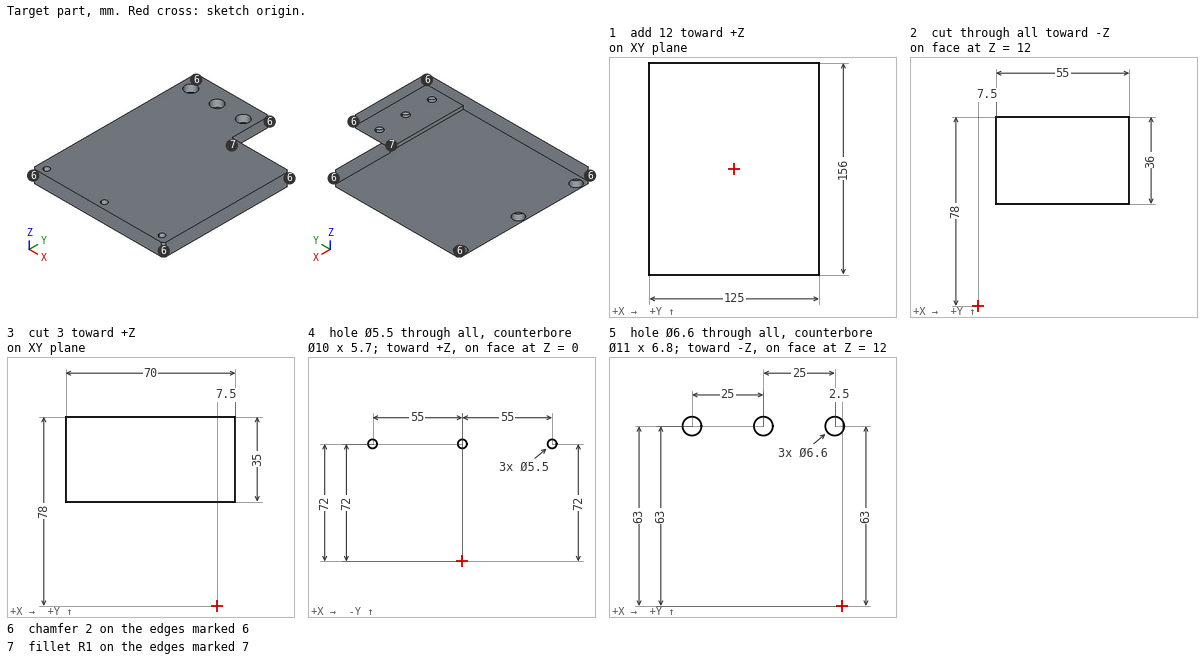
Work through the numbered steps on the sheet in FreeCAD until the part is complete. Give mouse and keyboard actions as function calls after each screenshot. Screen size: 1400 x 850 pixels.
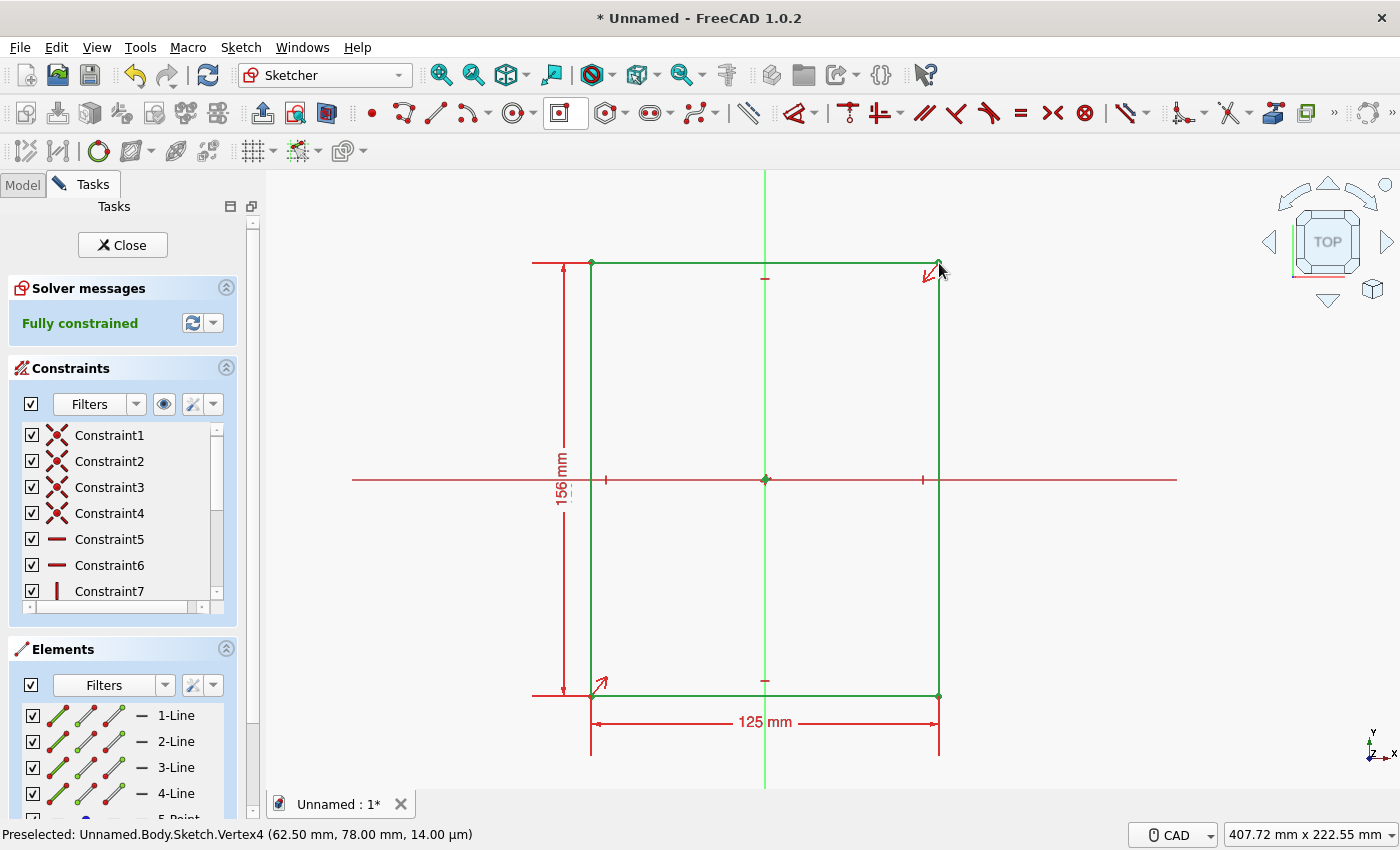
click(123, 245)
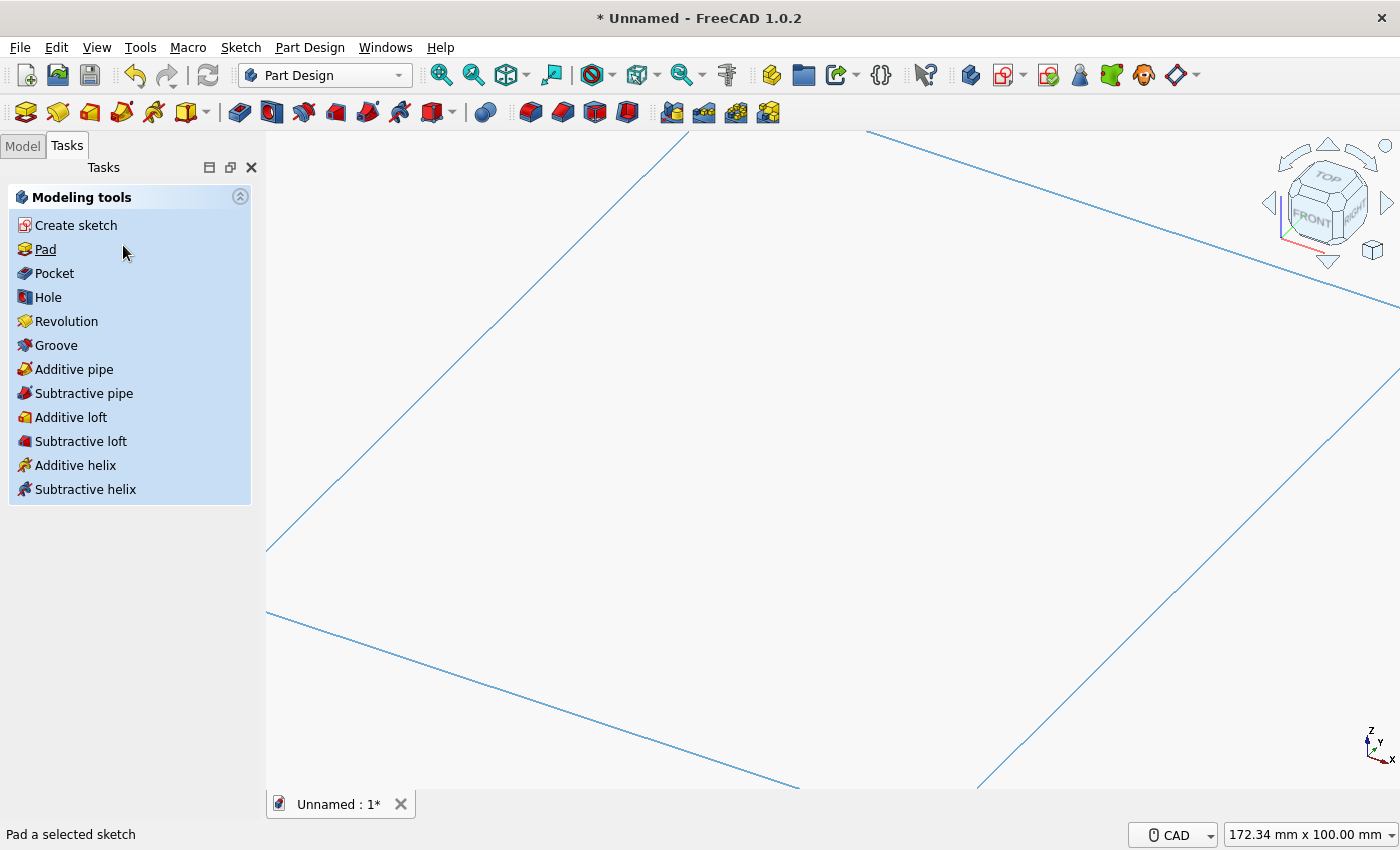
click(26, 112)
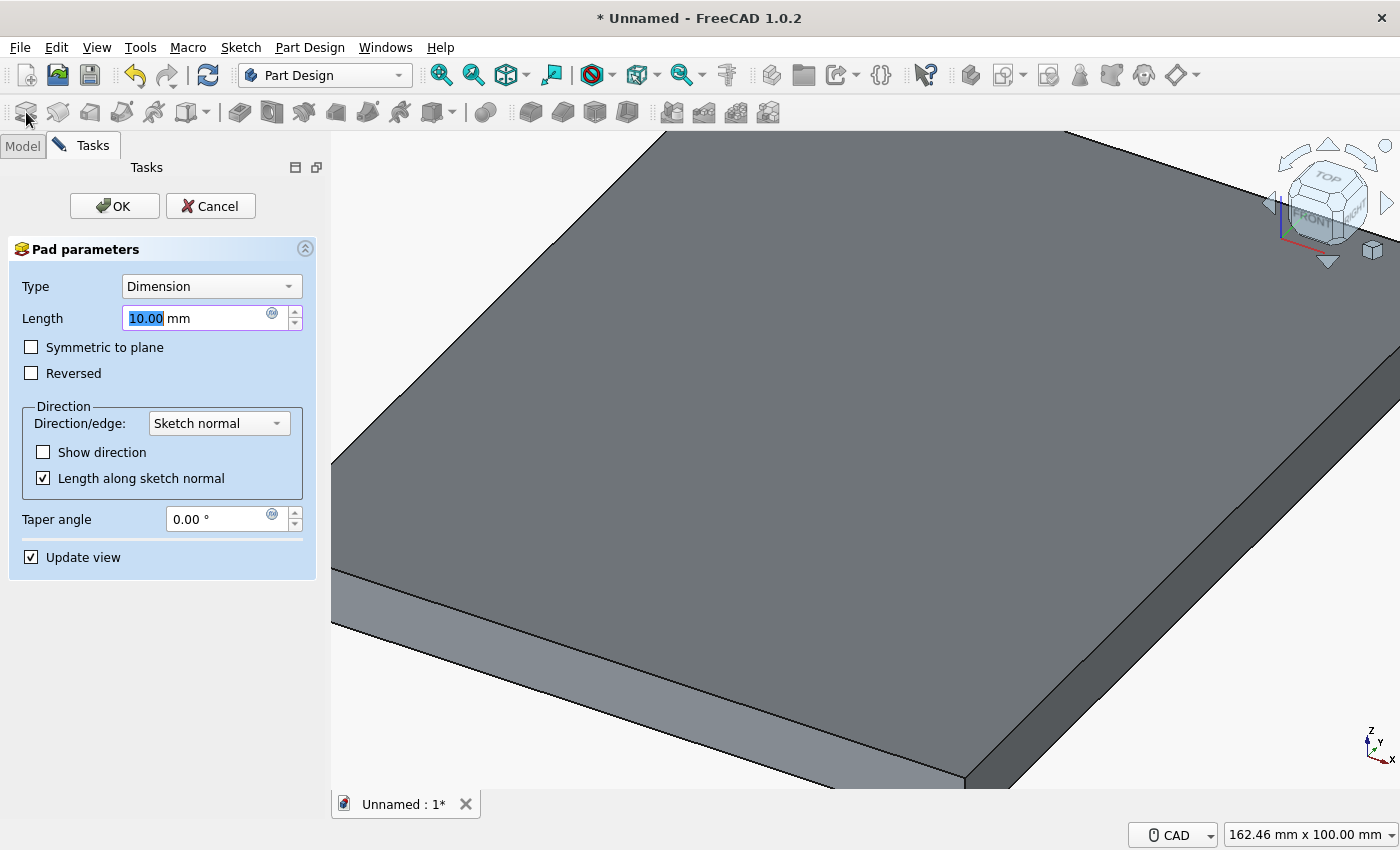
text(12)
key(Tab)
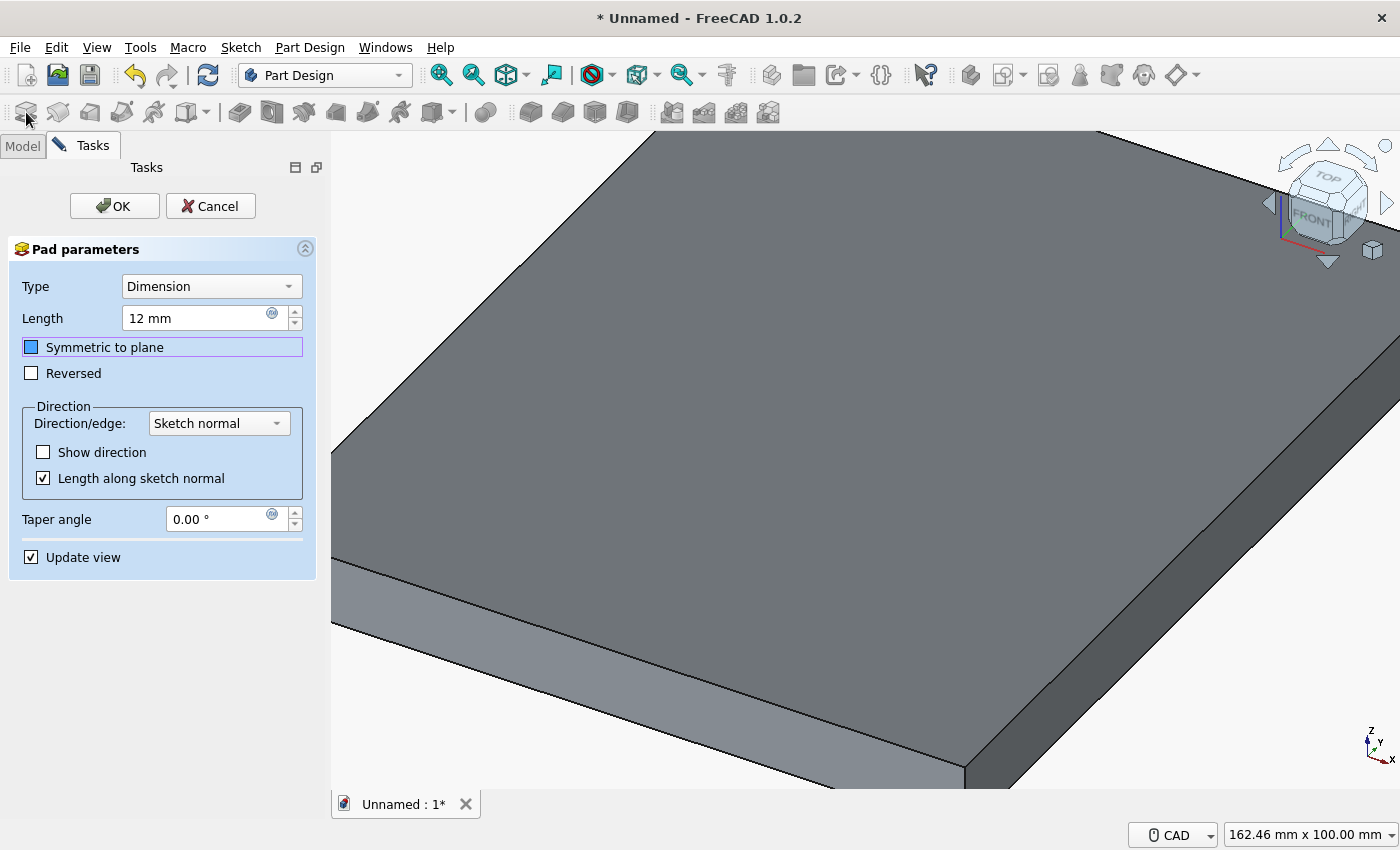
click(115, 206)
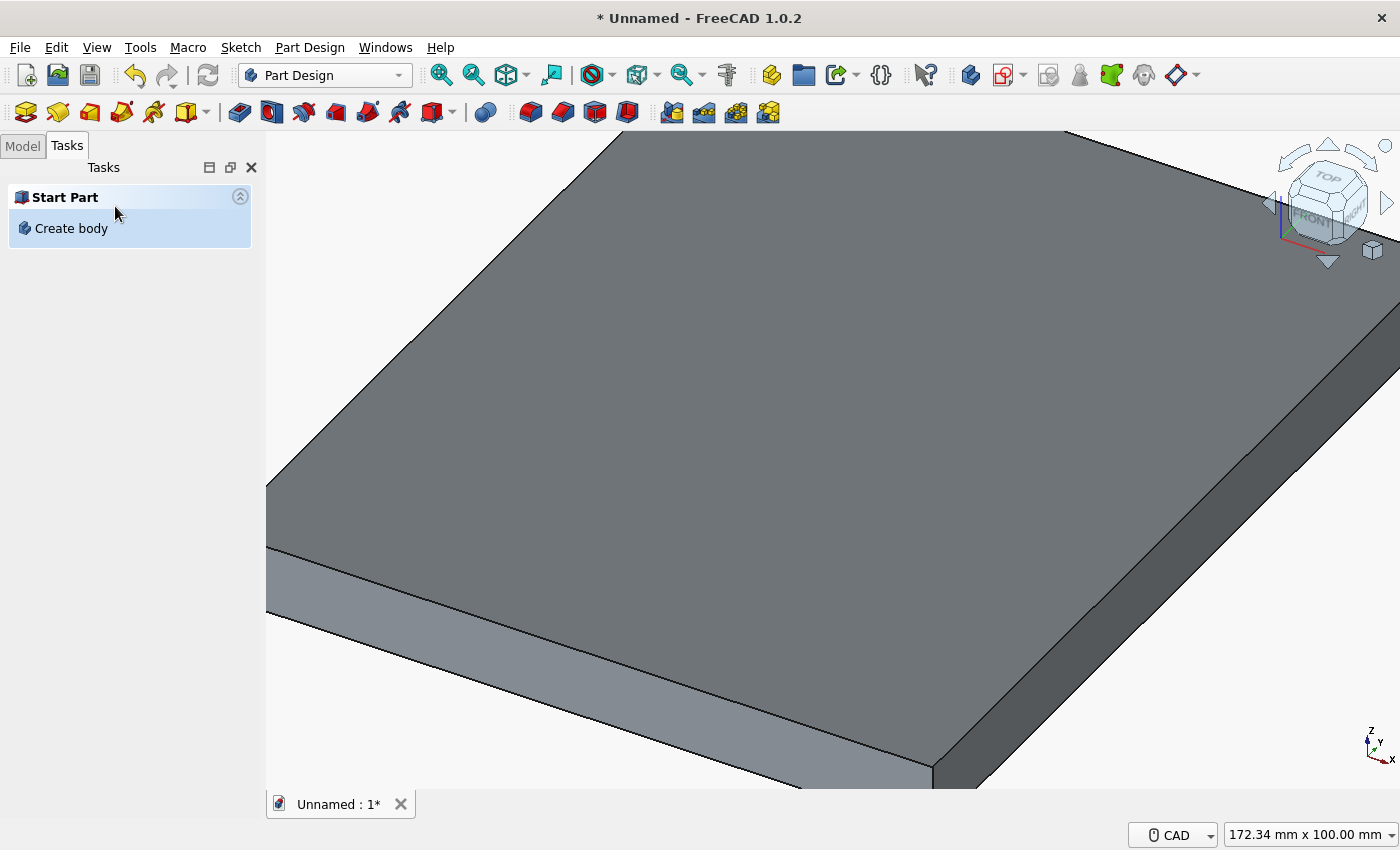
click(442, 76)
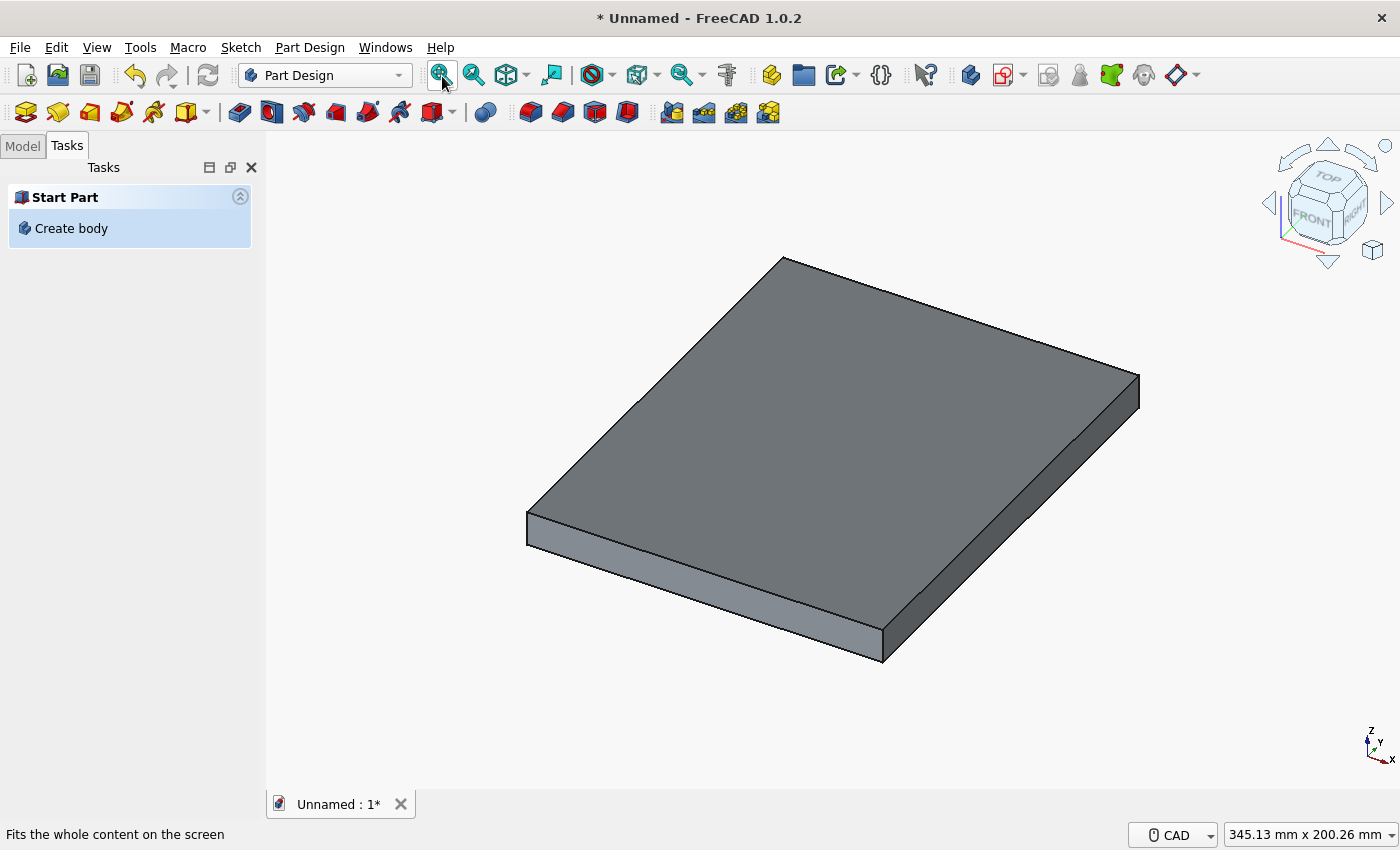
click(833, 443)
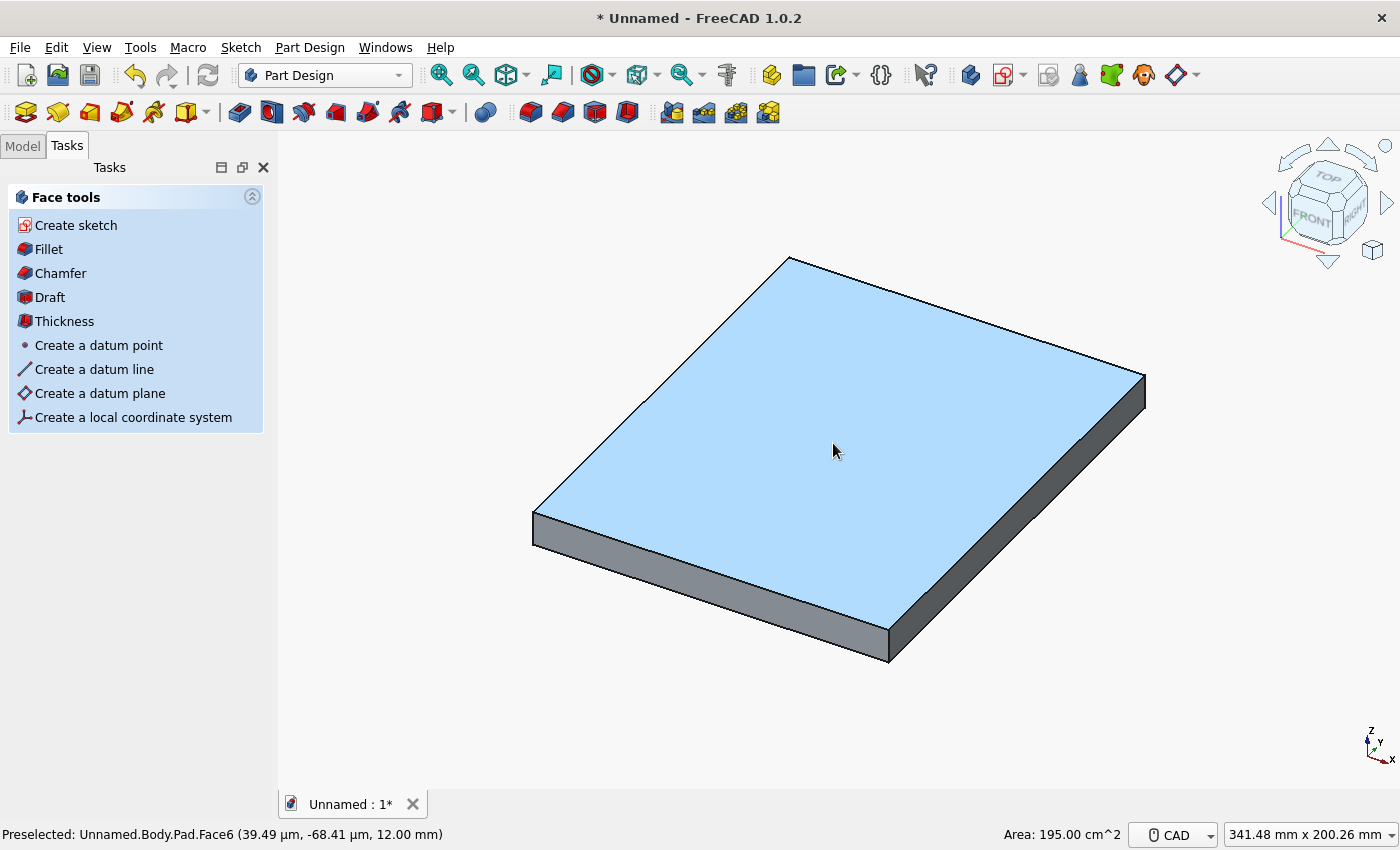
click(1004, 76)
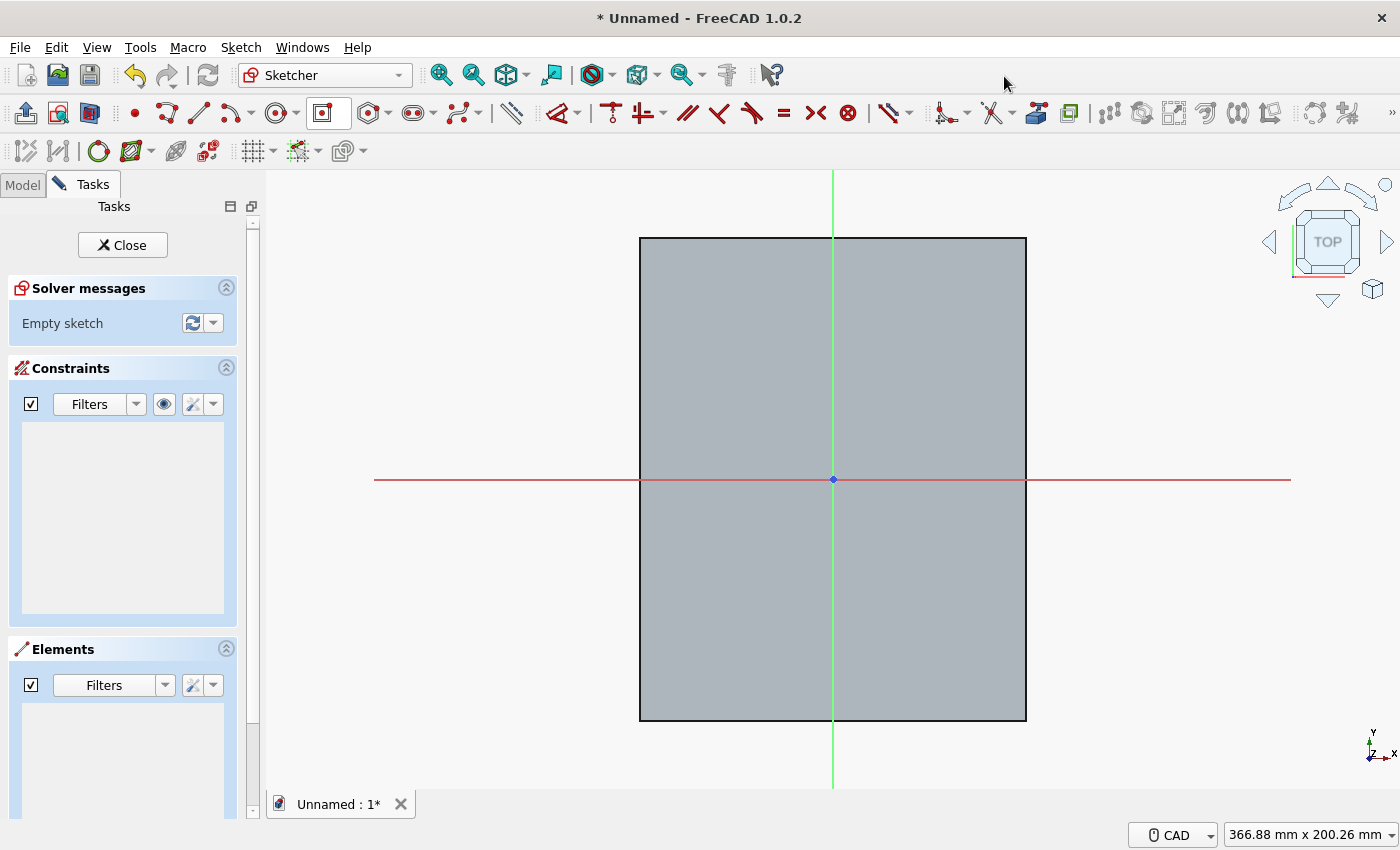
scroll(1235, 198, up, 2)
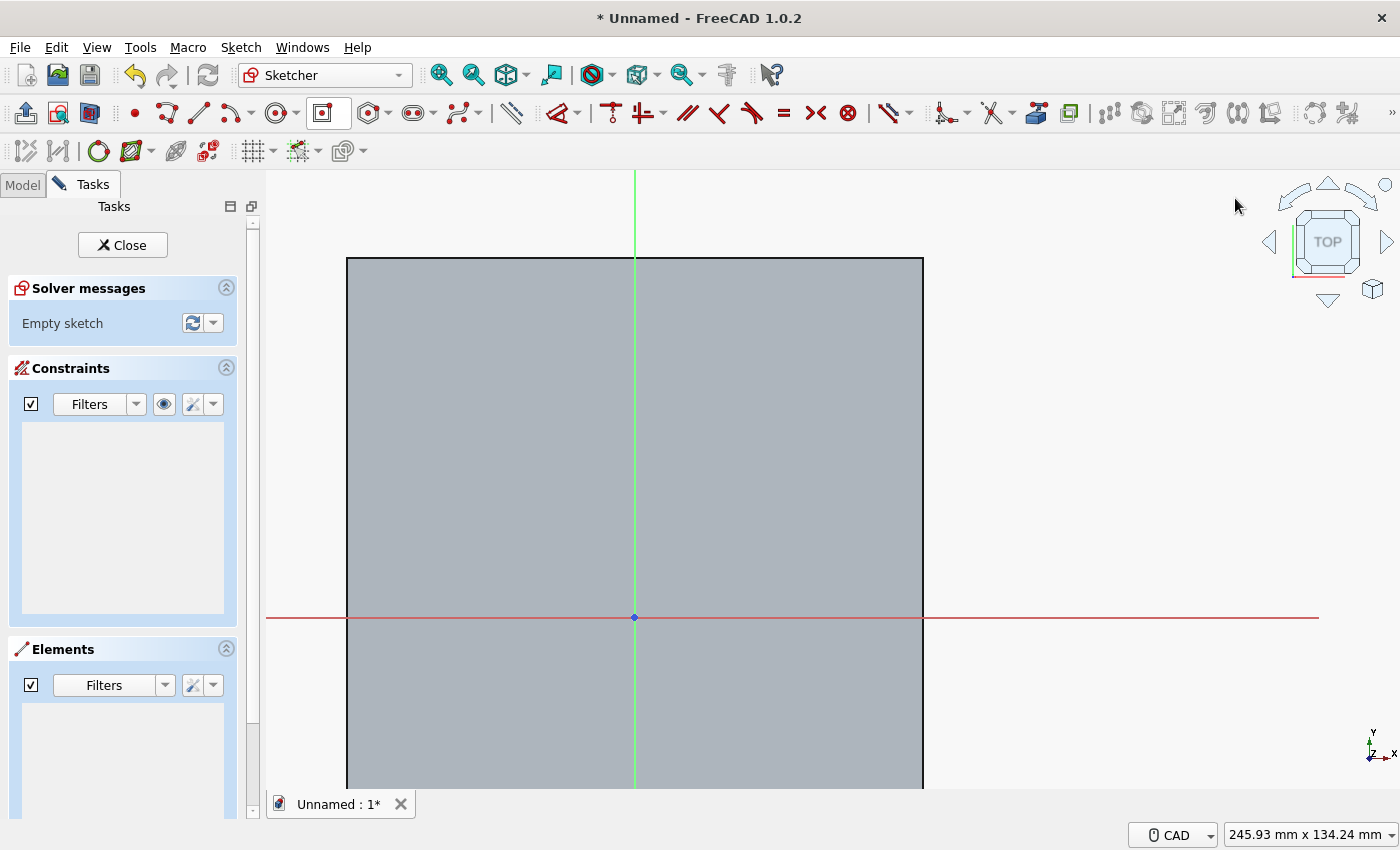
key(g)
key(r)